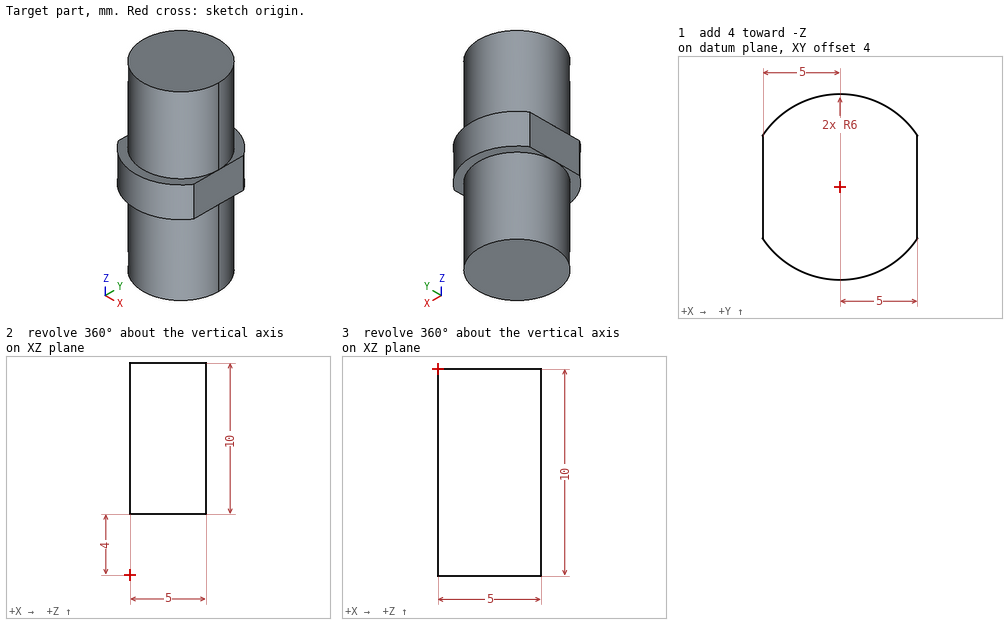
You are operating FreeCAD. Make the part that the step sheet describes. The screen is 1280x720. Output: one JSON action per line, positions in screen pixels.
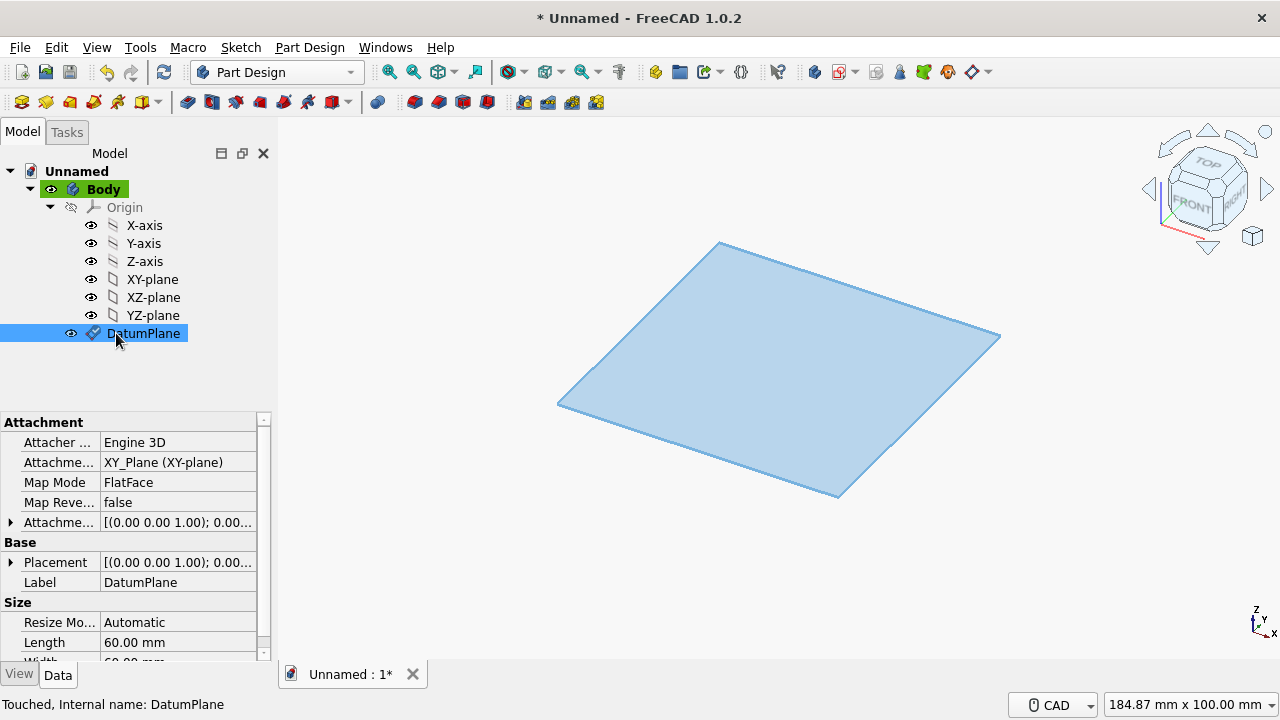
{"action": "left_click", "coordinate": [840, 72]}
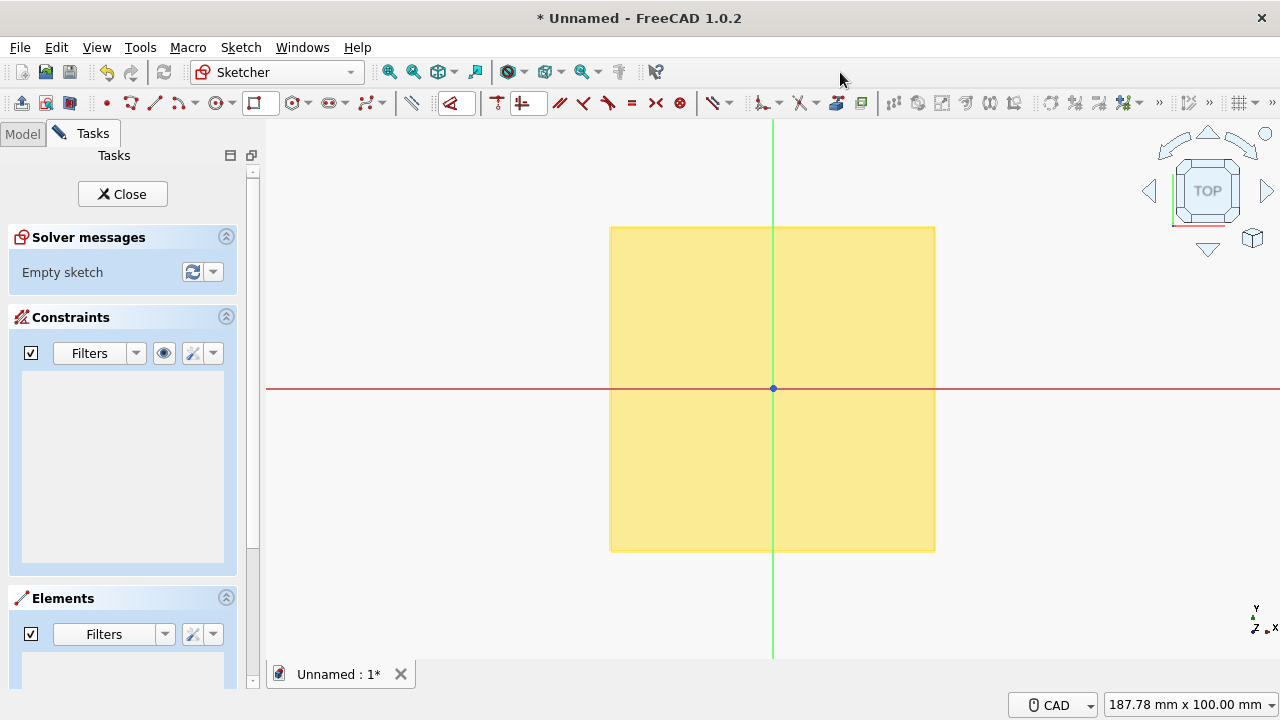
{"action": "scroll", "coordinate": [790, 389], "scroll_direction": "up", "scroll_amount": 8}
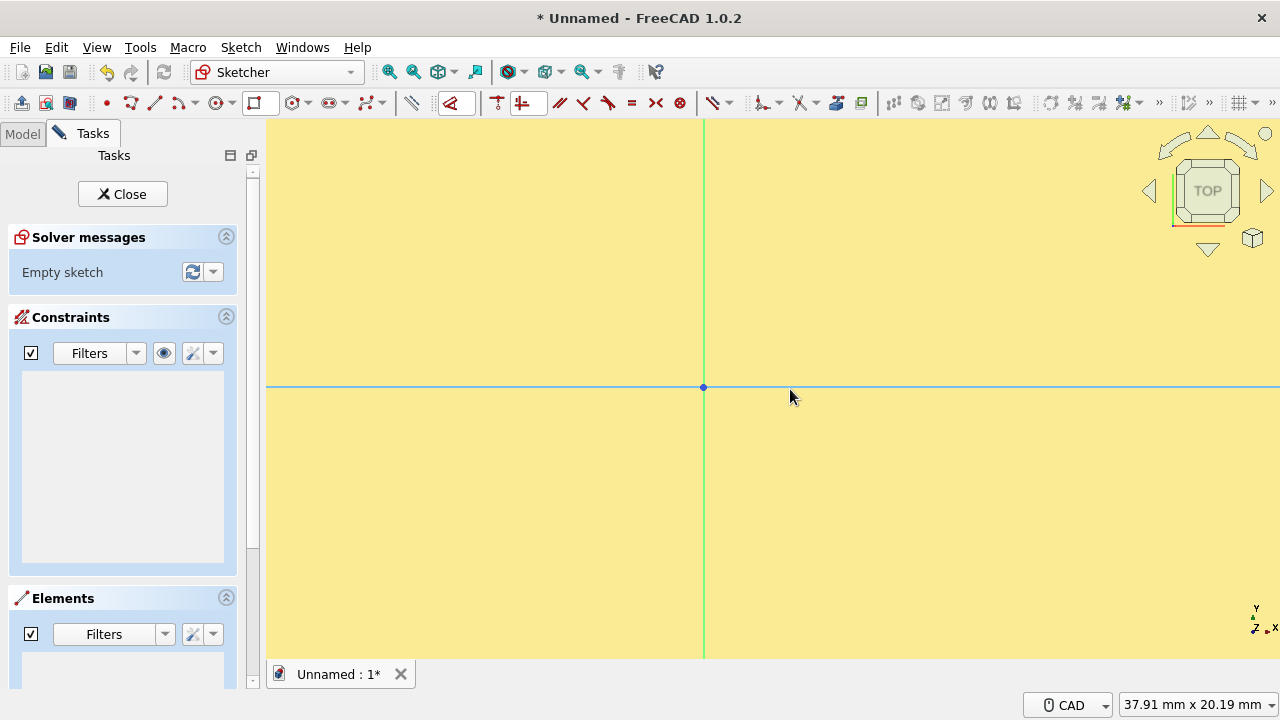
{"action": "left_click", "coordinate": [156, 104]}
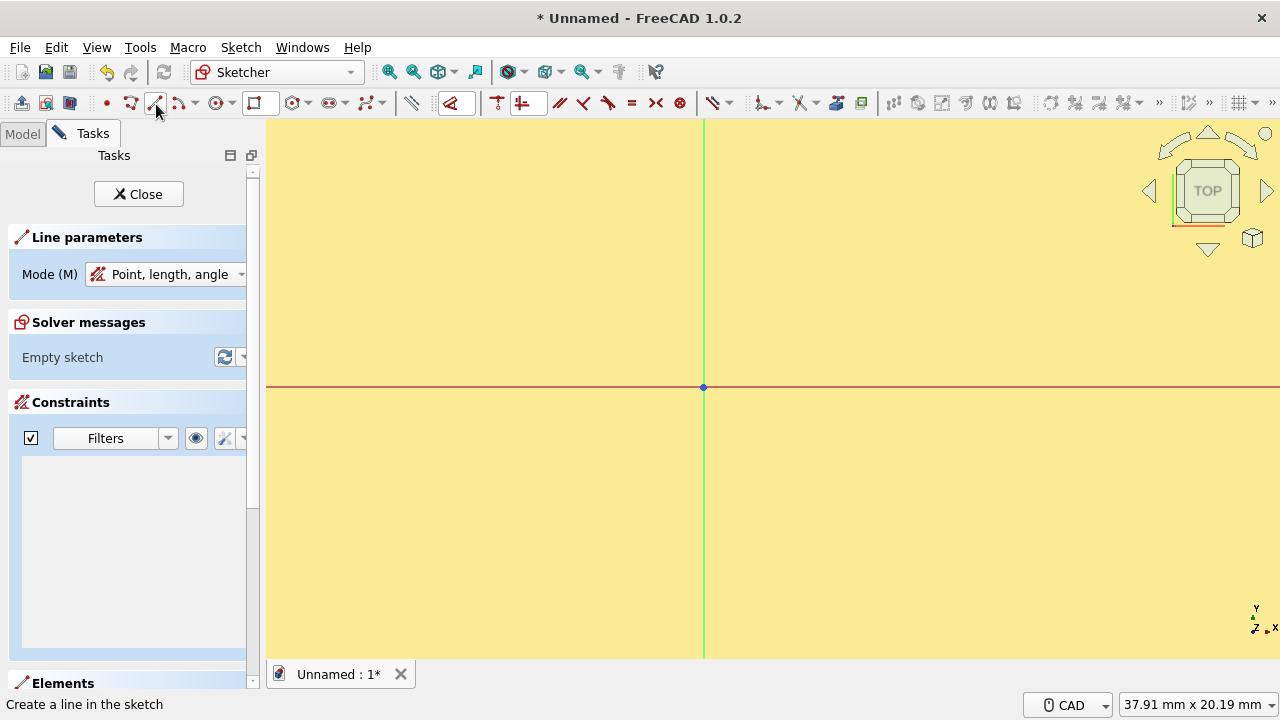
{"action": "left_click", "coordinate": [837, 476]}
{"action": "left_click", "coordinate": [837, 298]}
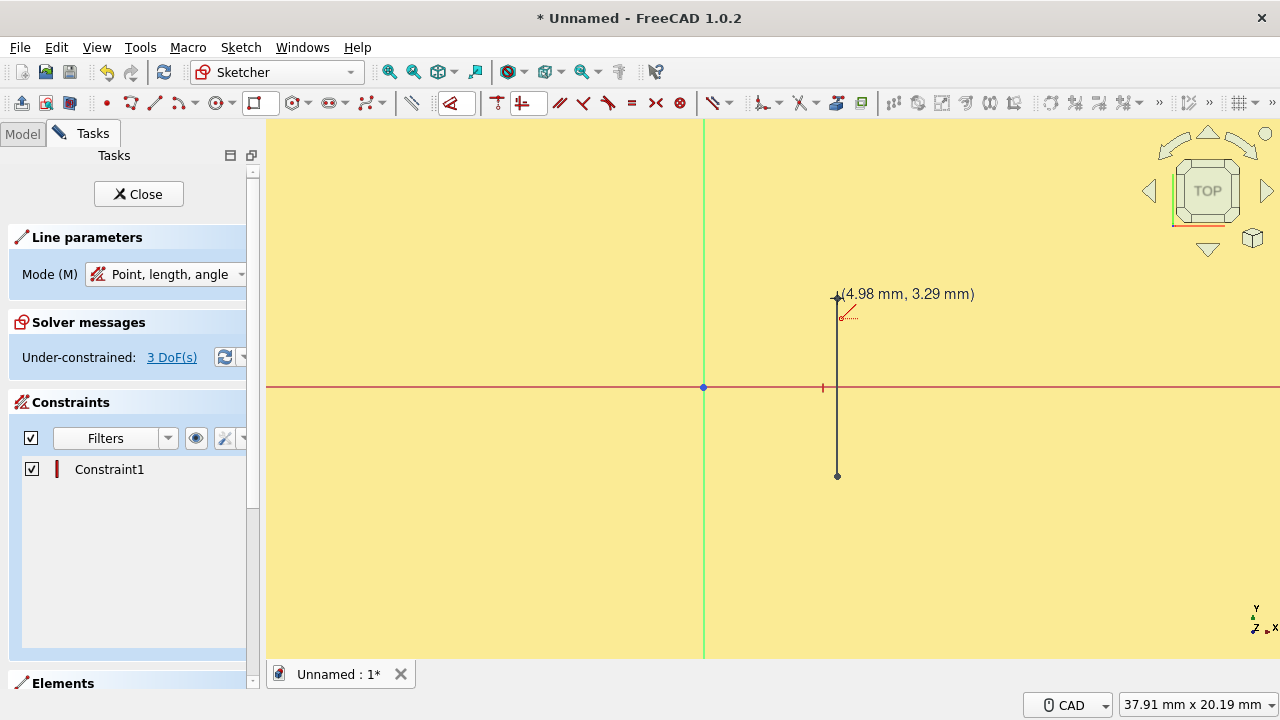
{"action": "left_click", "coordinate": [570, 298]}
{"action": "left_click", "coordinate": [570, 476]}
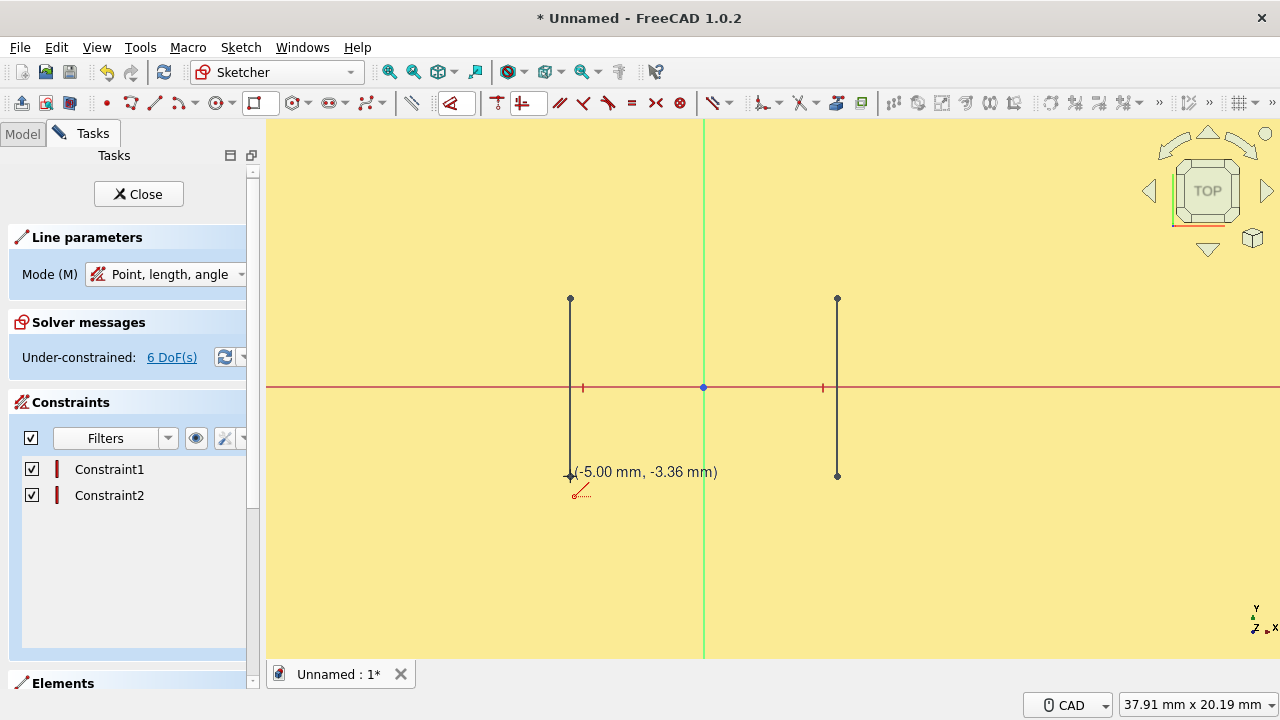
{"action": "left_click", "coordinate": [198, 104]}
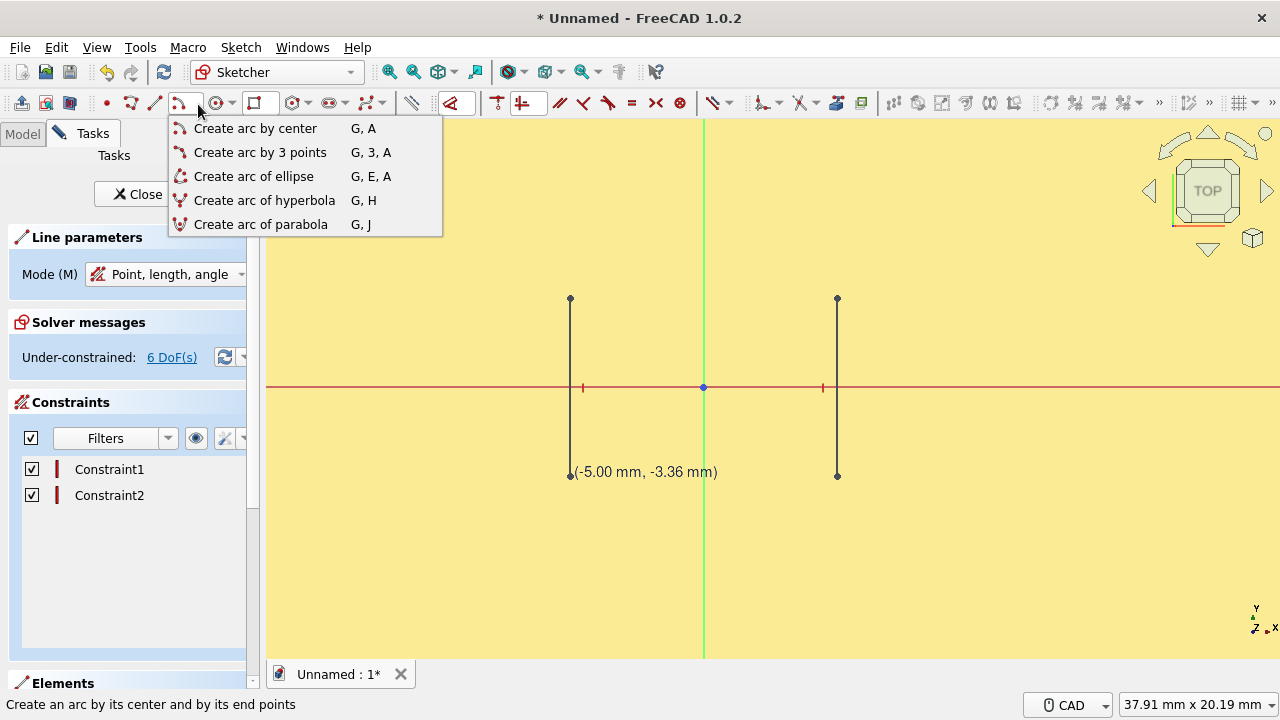
{"action": "left_click", "coordinate": [306, 152]}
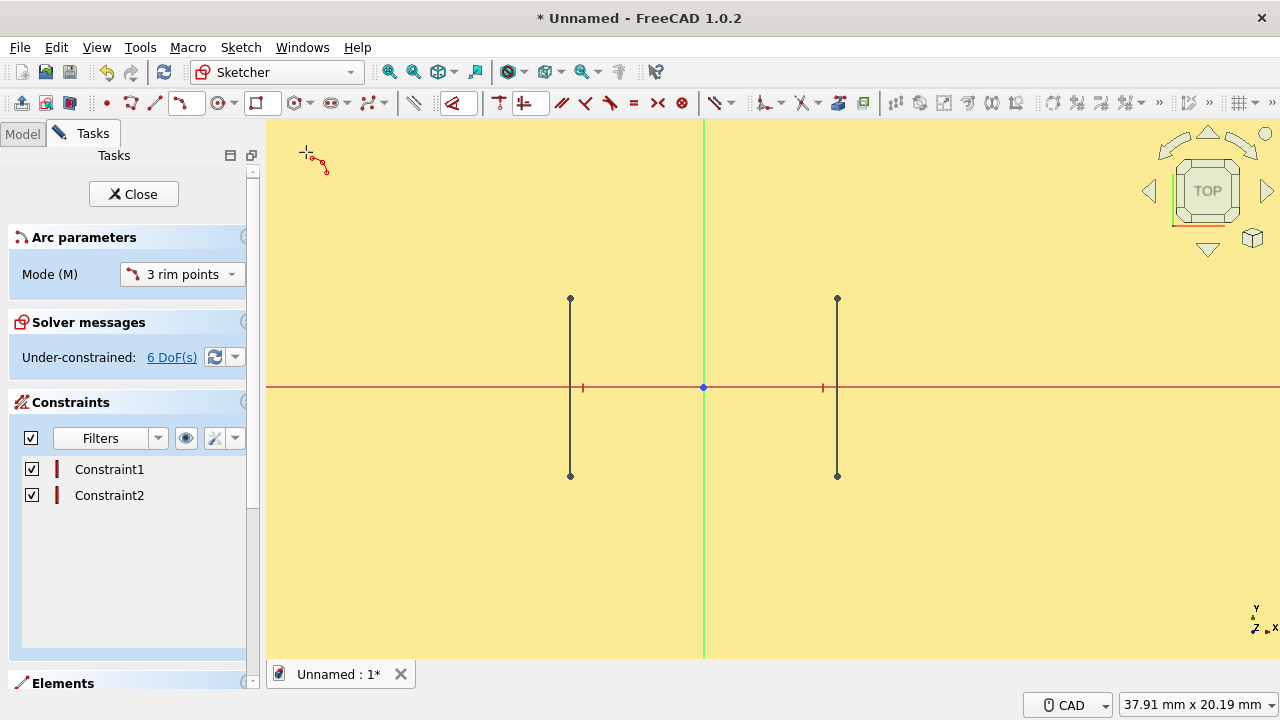
{"action": "left_click", "coordinate": [837, 299]}
{"action": "left_click", "coordinate": [570, 299]}
{"action": "left_click", "coordinate": [735, 230]}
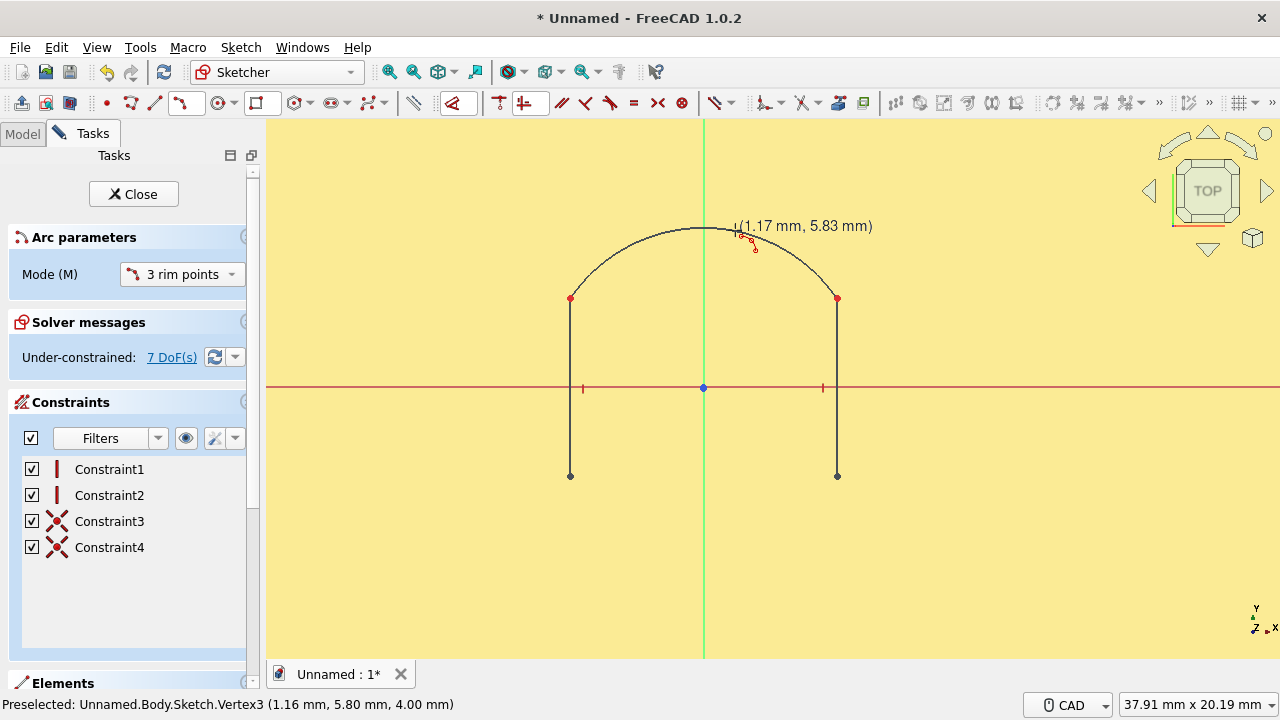
{"action": "left_click", "coordinate": [570, 477]}
{"action": "left_click", "coordinate": [837, 477]}
{"action": "left_click", "coordinate": [672, 544]}
{"action": "key", "text": "Escape"}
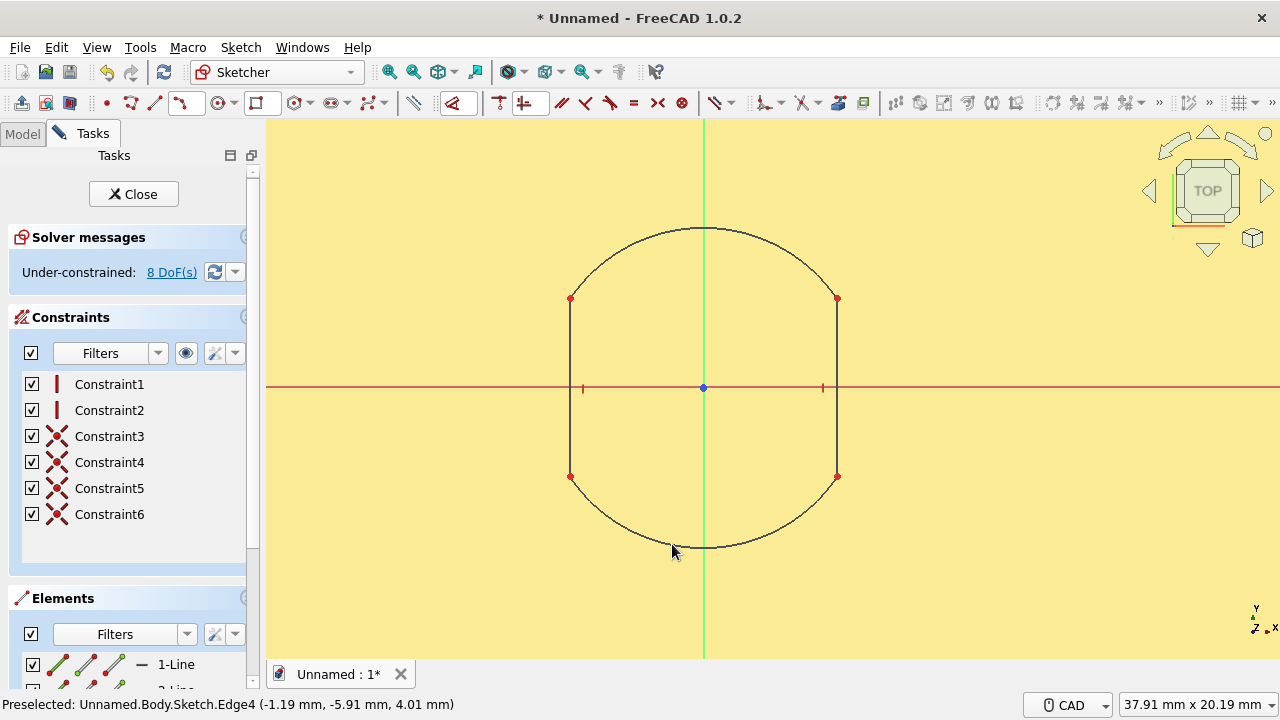
{"action": "left_click", "coordinate": [765, 240]}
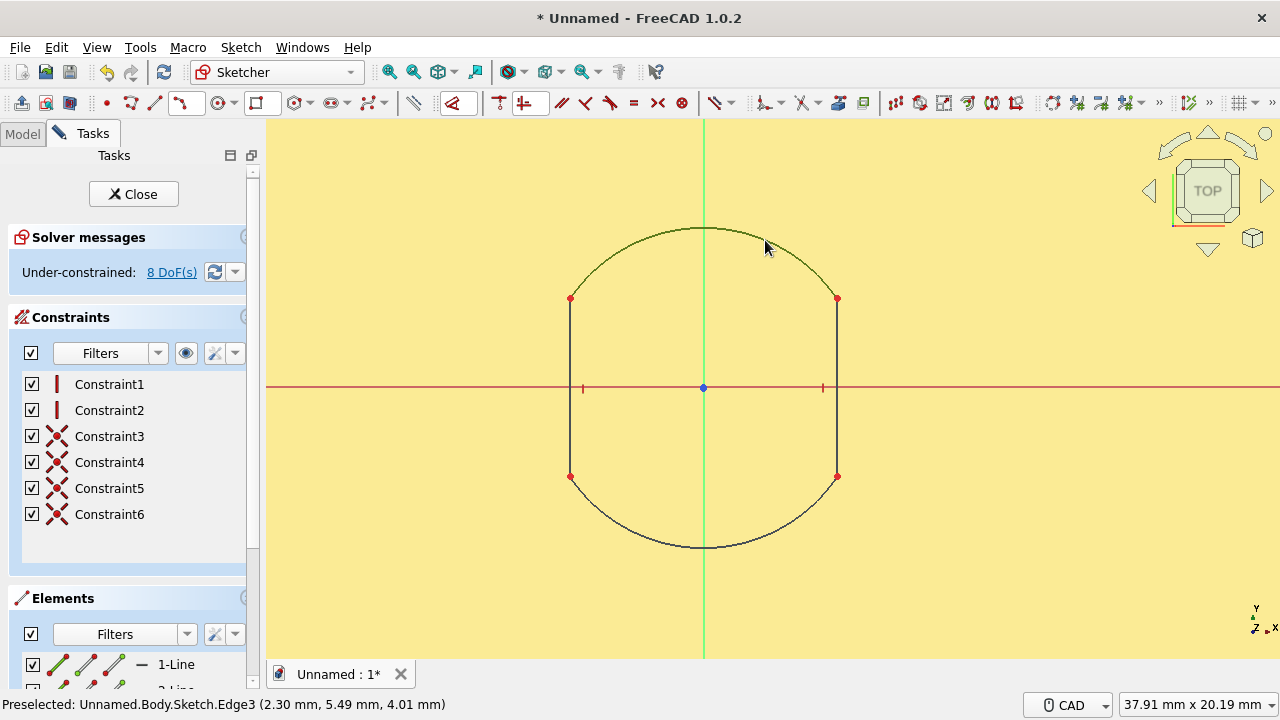
{"action": "left_click", "coordinate": [642, 536]}